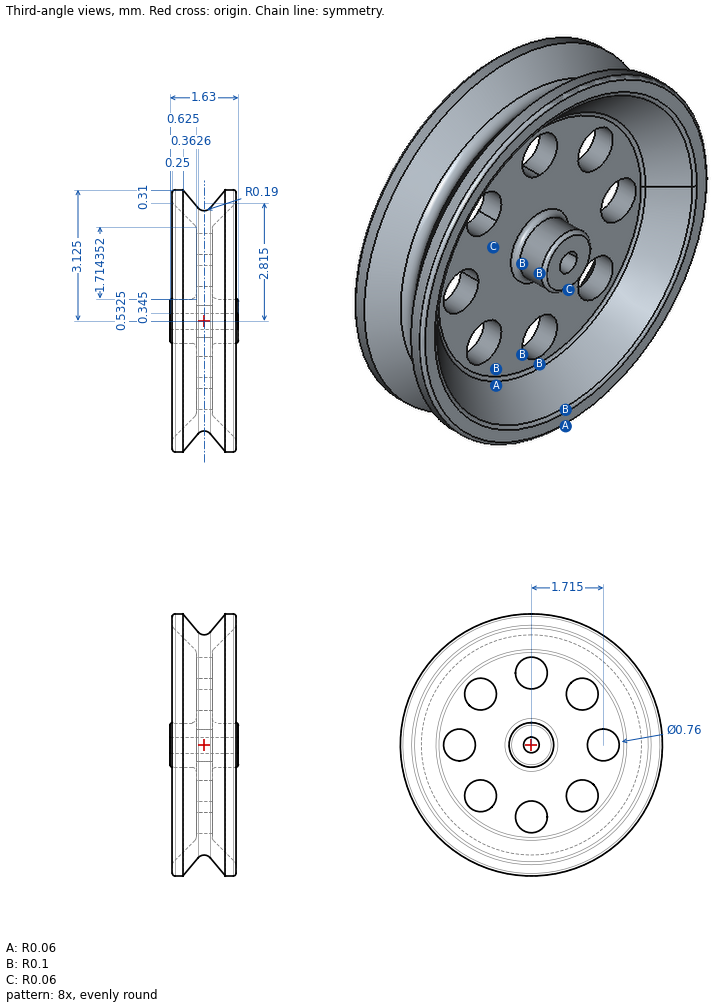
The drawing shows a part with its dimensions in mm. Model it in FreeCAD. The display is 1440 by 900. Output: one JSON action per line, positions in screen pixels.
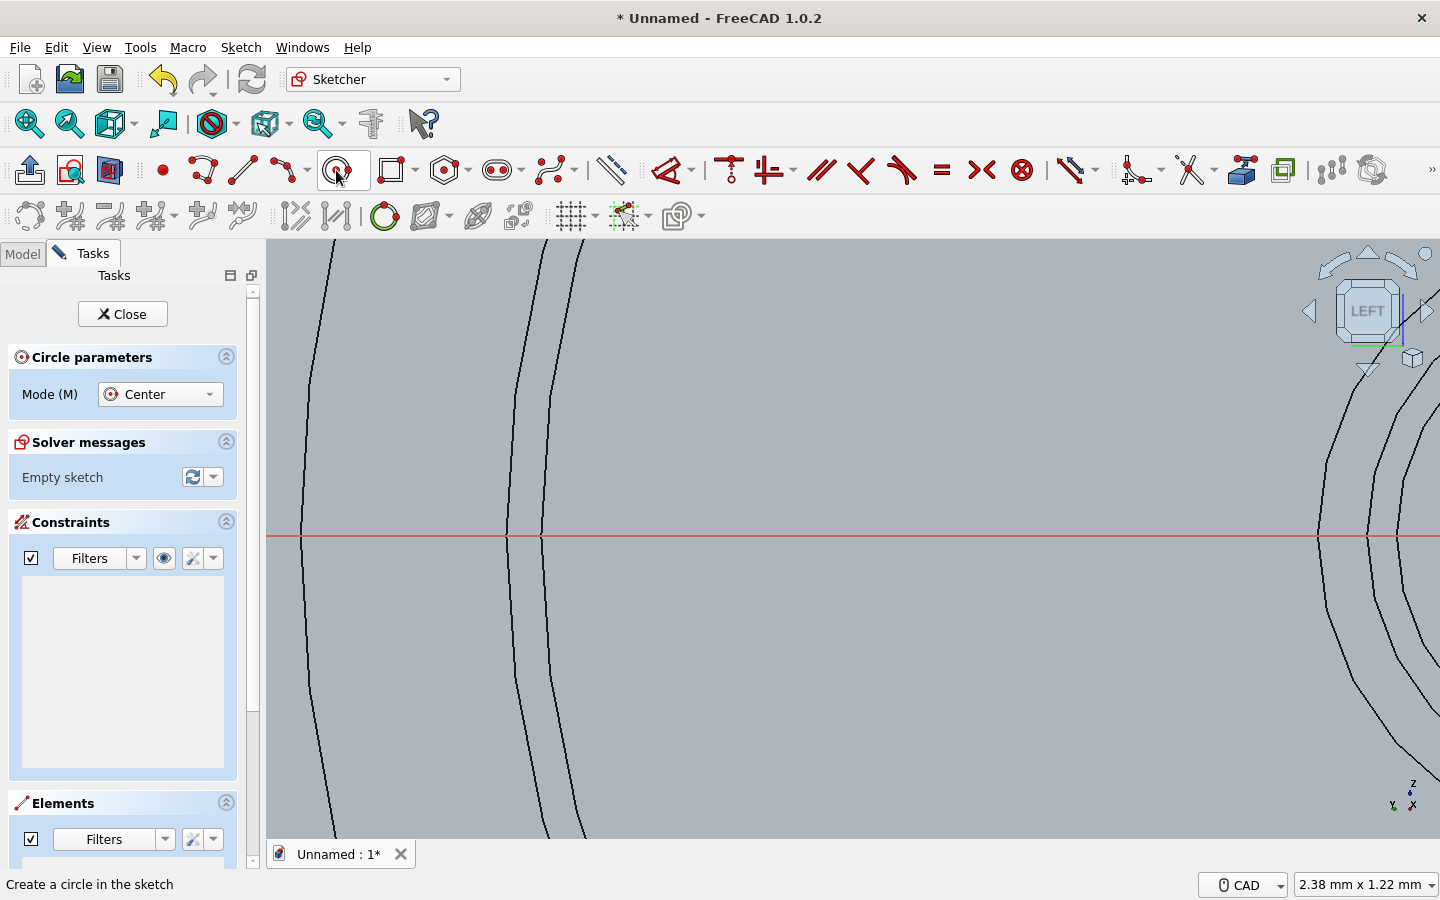
{"action": "left_click", "coordinate": [783, 536]}
{"action": "left_click", "coordinate": [916, 403]}
{"action": "key", "text": "Escape"}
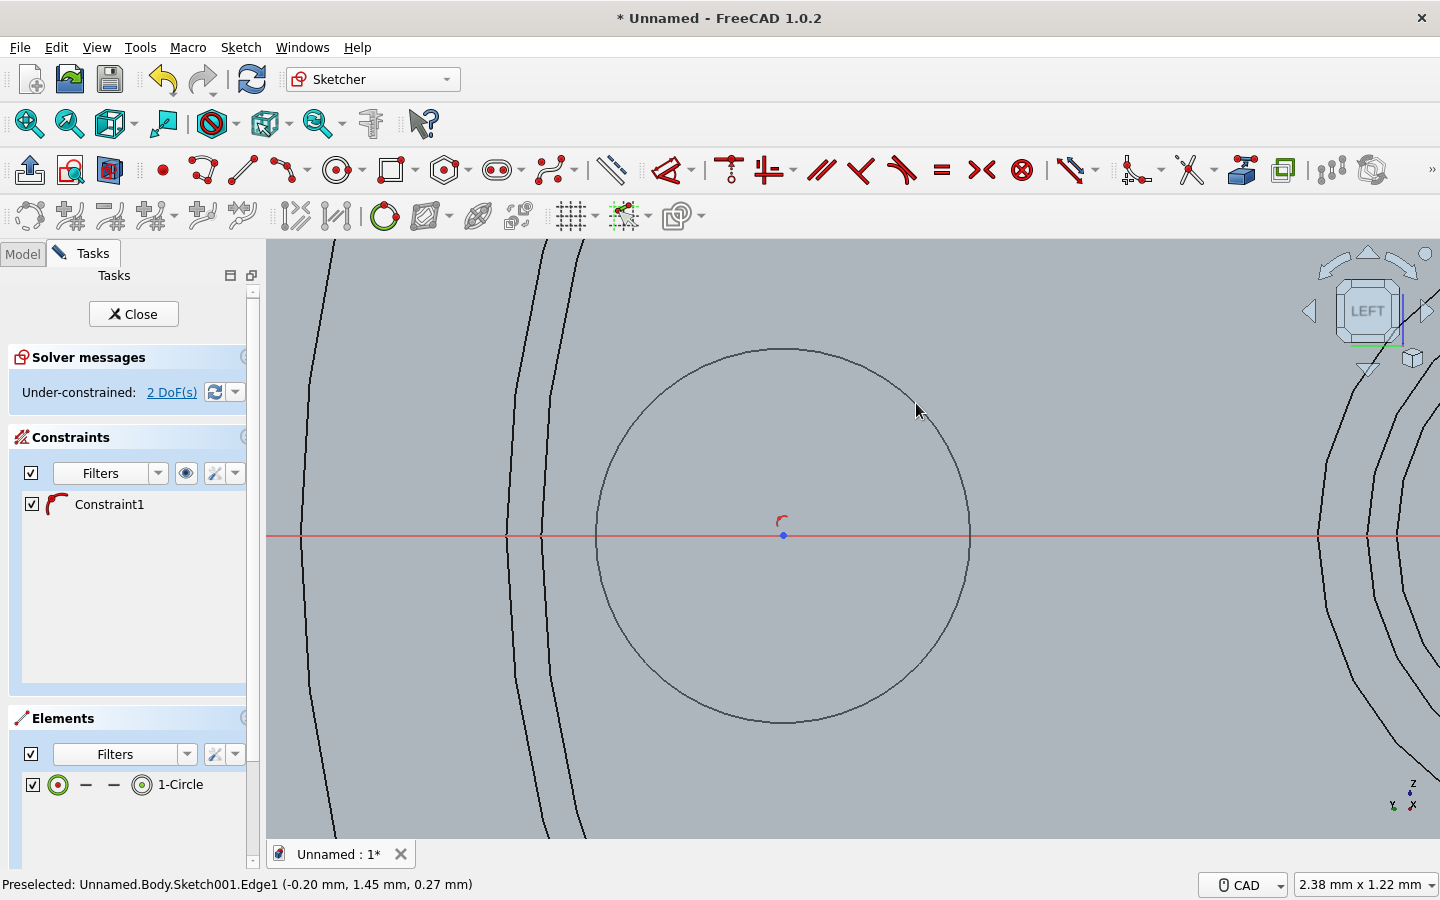
{"action": "left_click", "coordinate": [666, 170]}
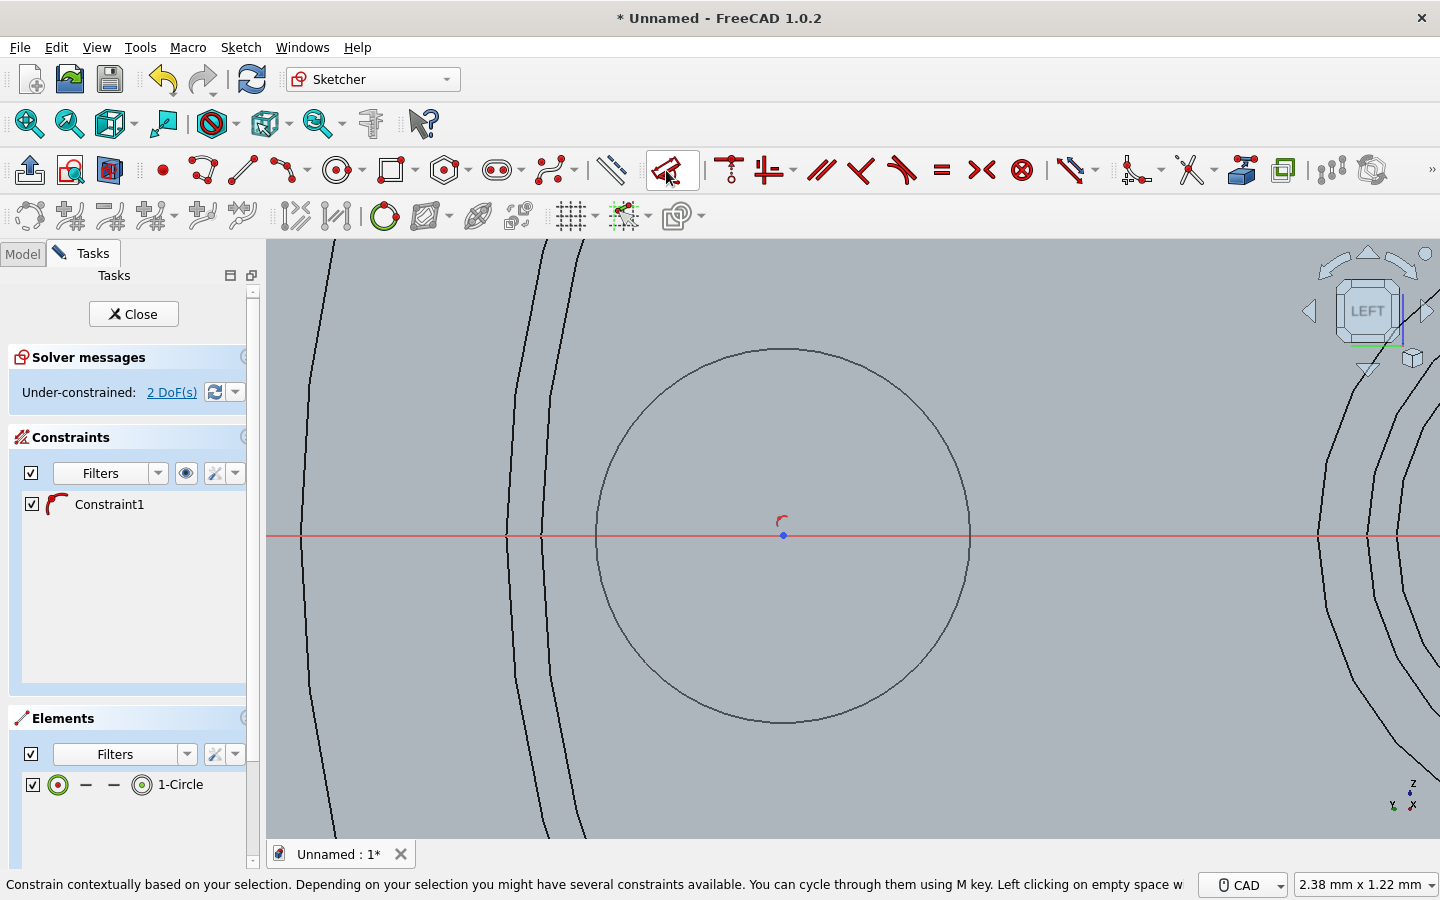
{"action": "left_click", "coordinate": [915, 403]}
{"action": "left_click", "coordinate": [938, 380]}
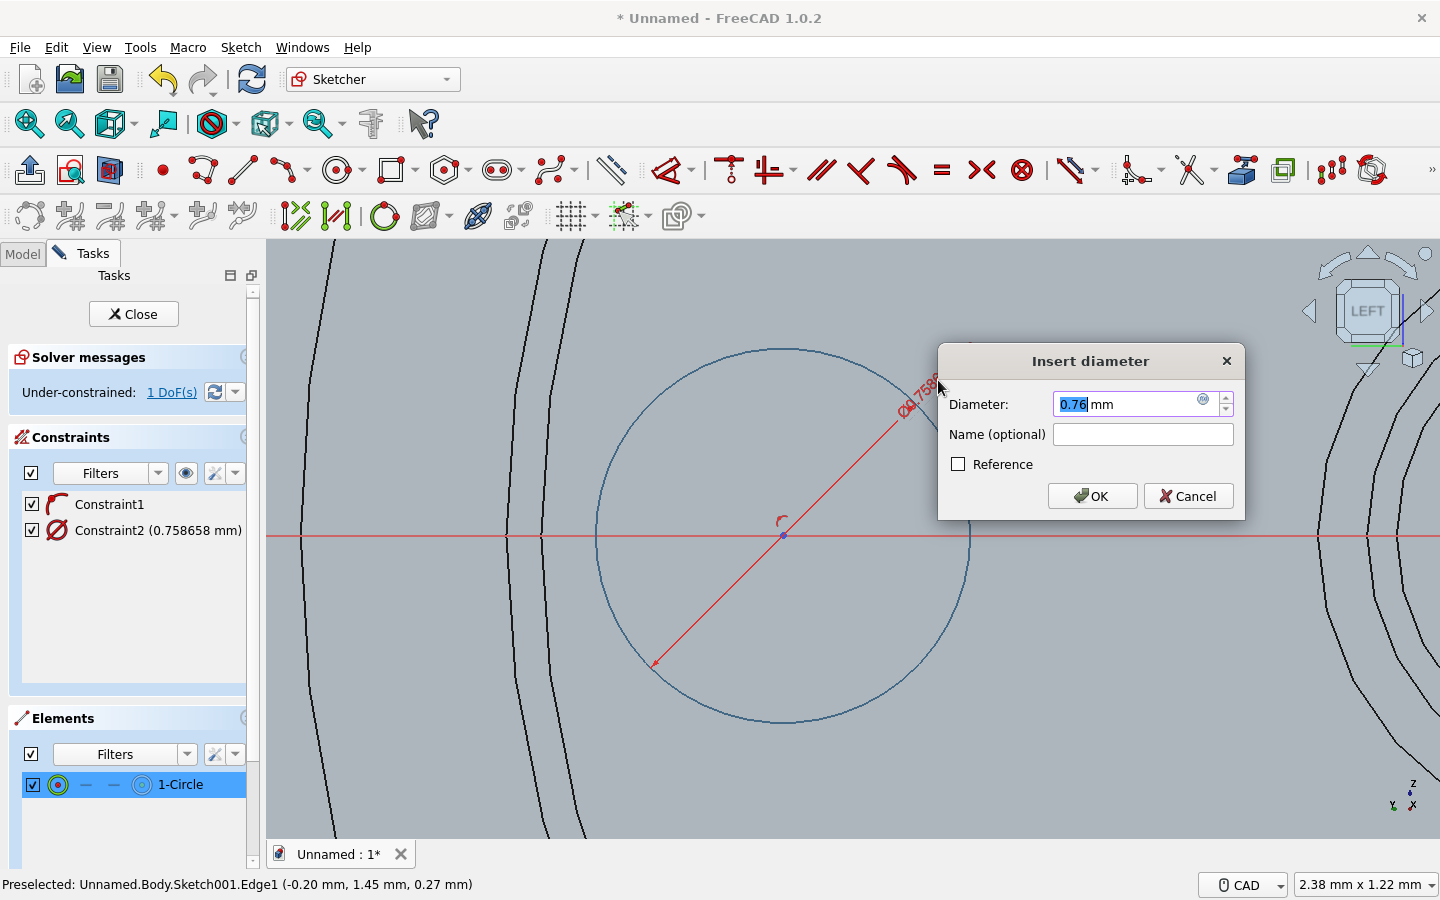
{"action": "type", "text": "0.76"}
{"action": "key", "text": "Return"}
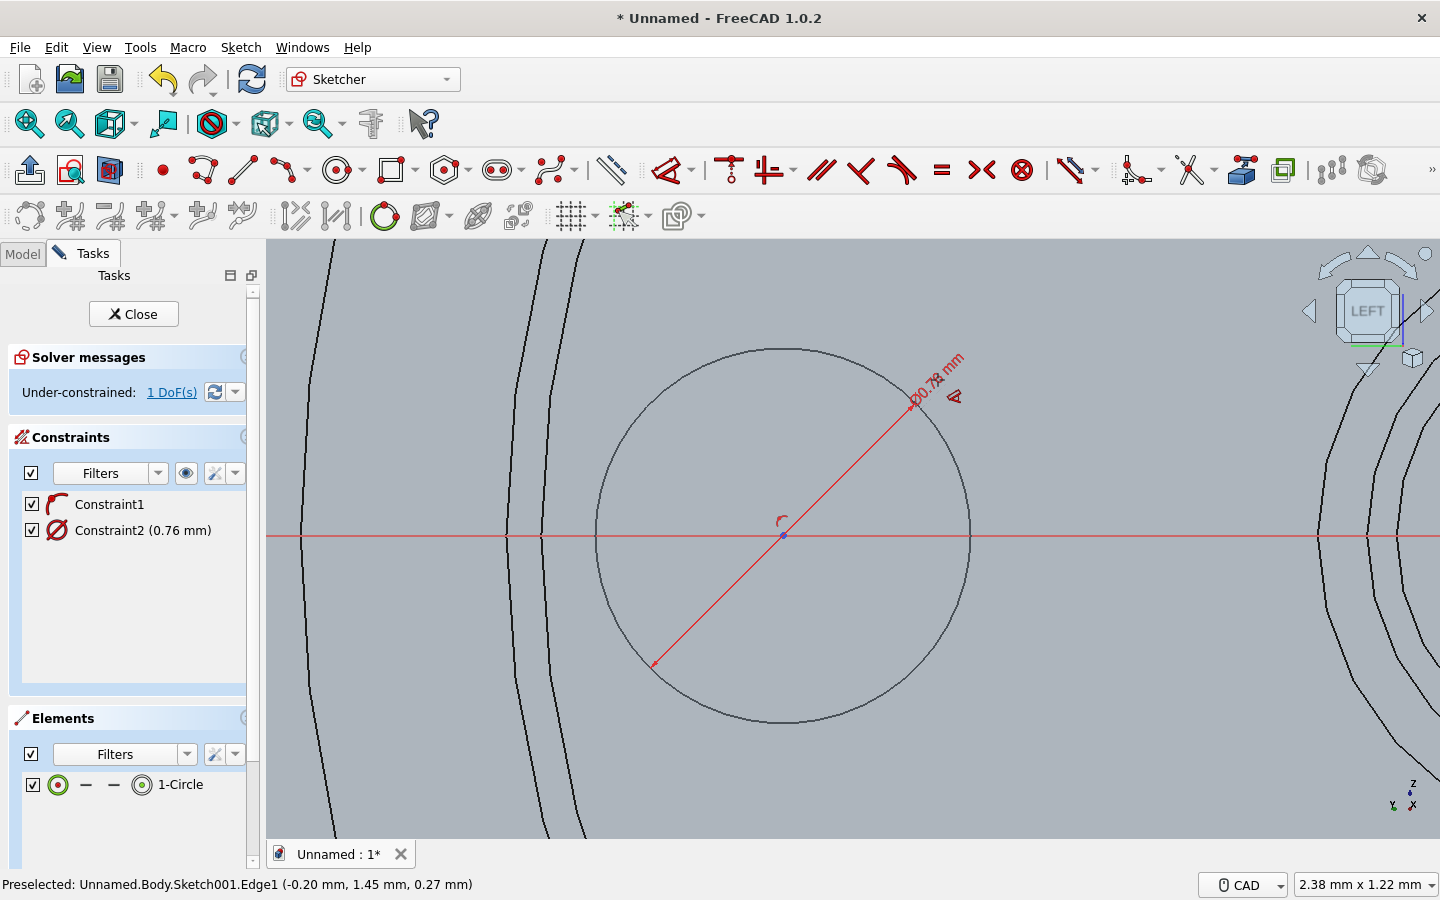
{"action": "left_click", "coordinate": [783, 536]}
{"action": "left_click", "coordinate": [1029, 570]}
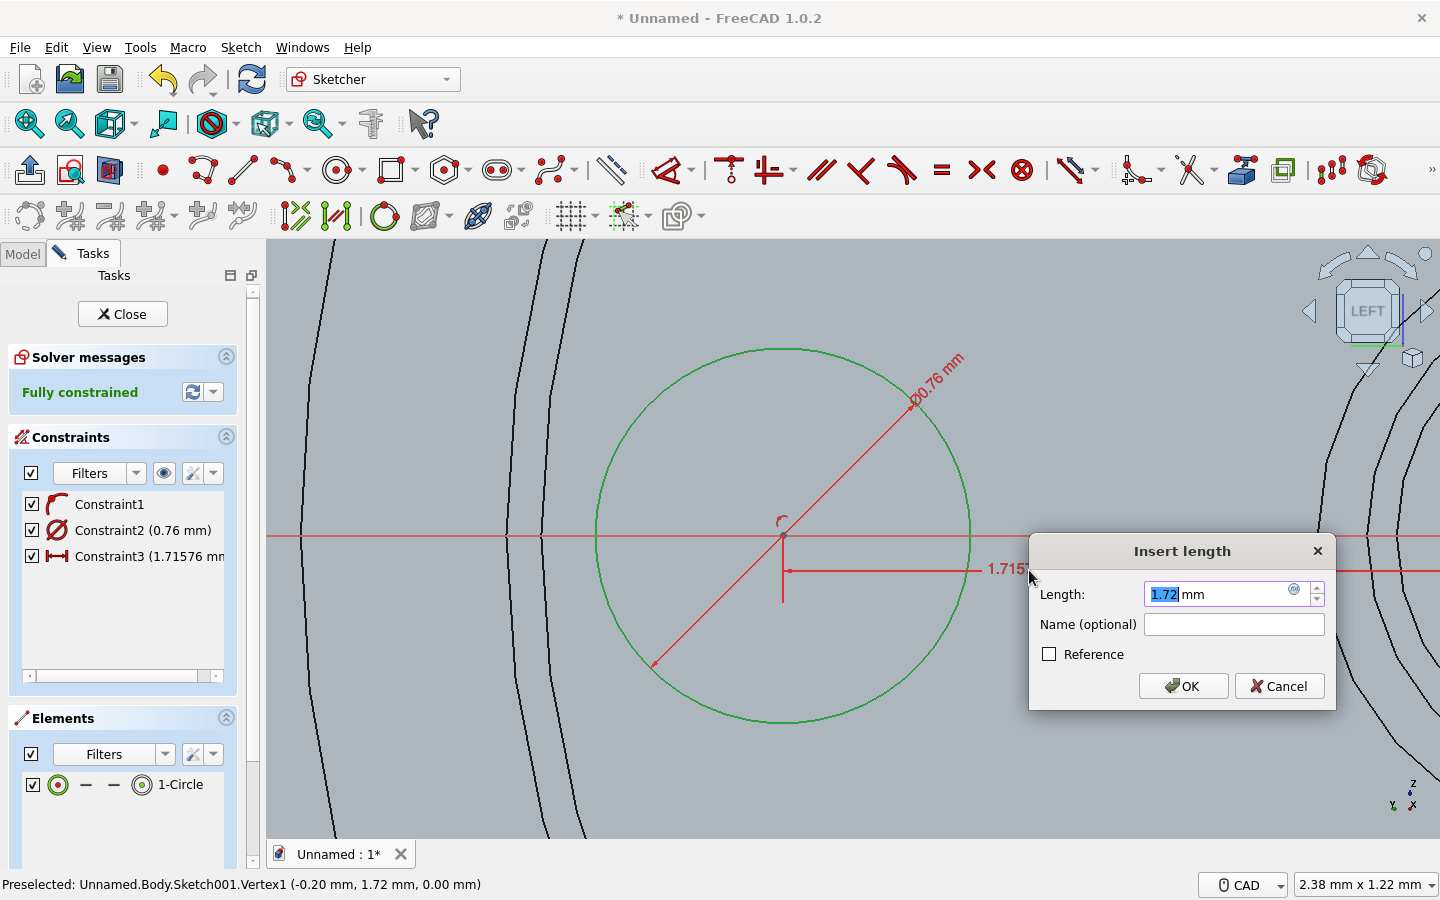
{"action": "type", "text": "1.715"}
{"action": "key", "text": "Return"}
{"action": "key", "text": "Escape"}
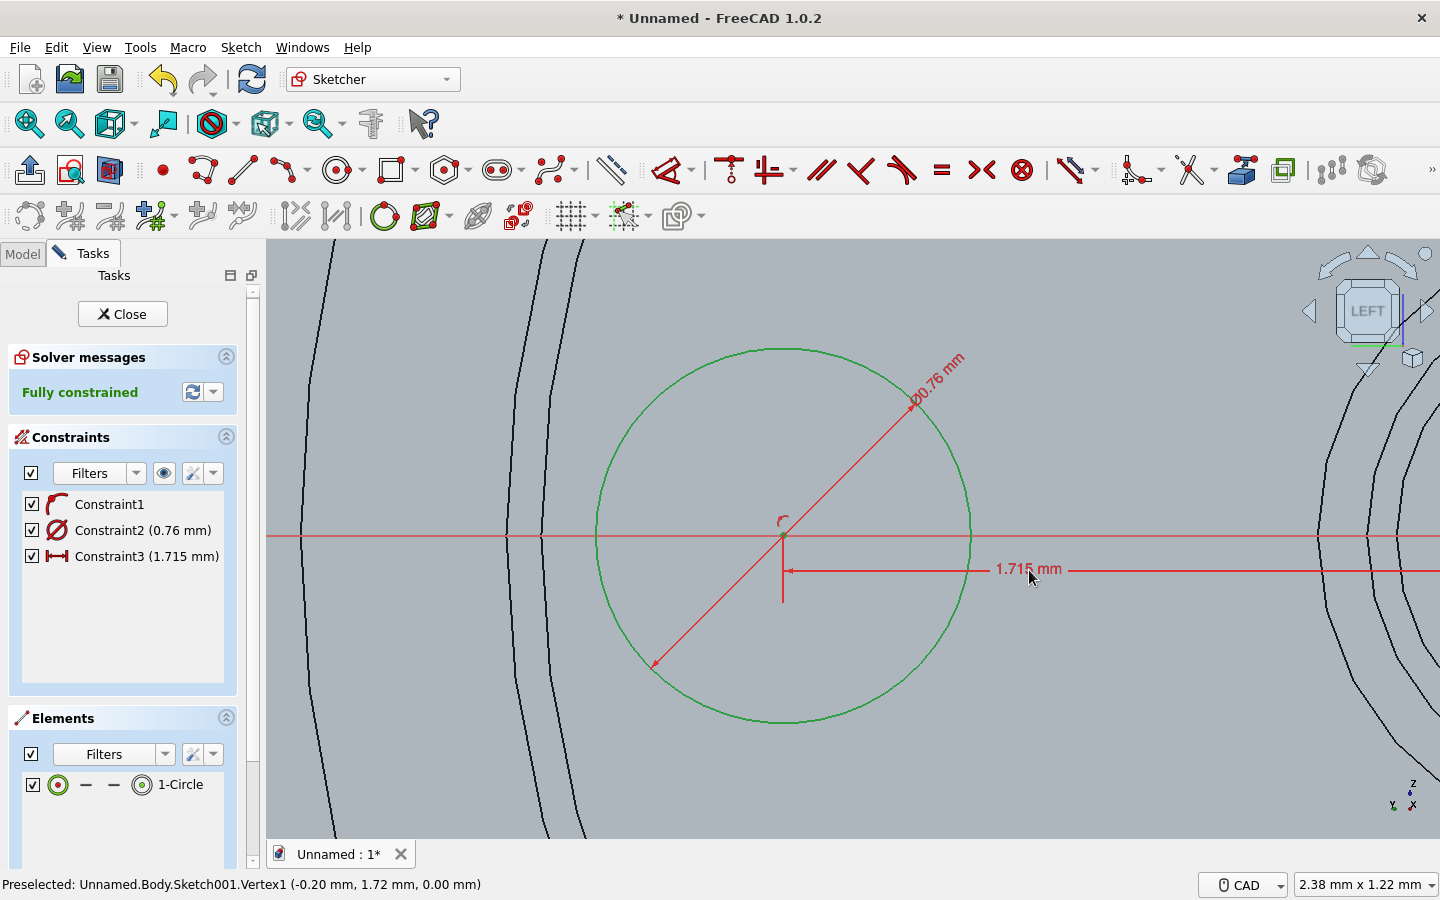
{"action": "left_click", "coordinate": [123, 314]}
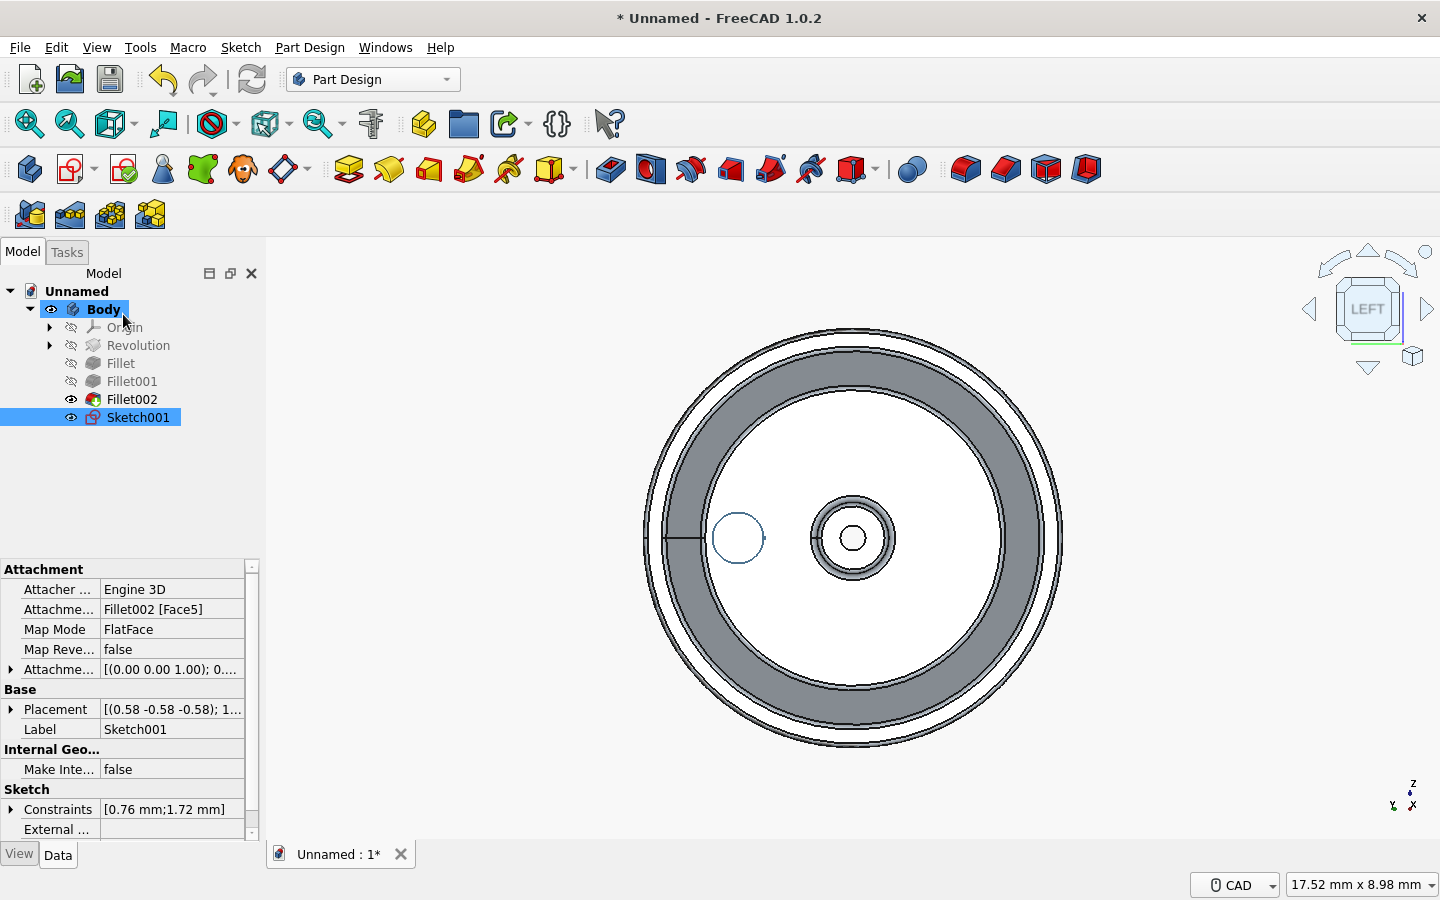
{"action": "left_click", "coordinate": [612, 170]}